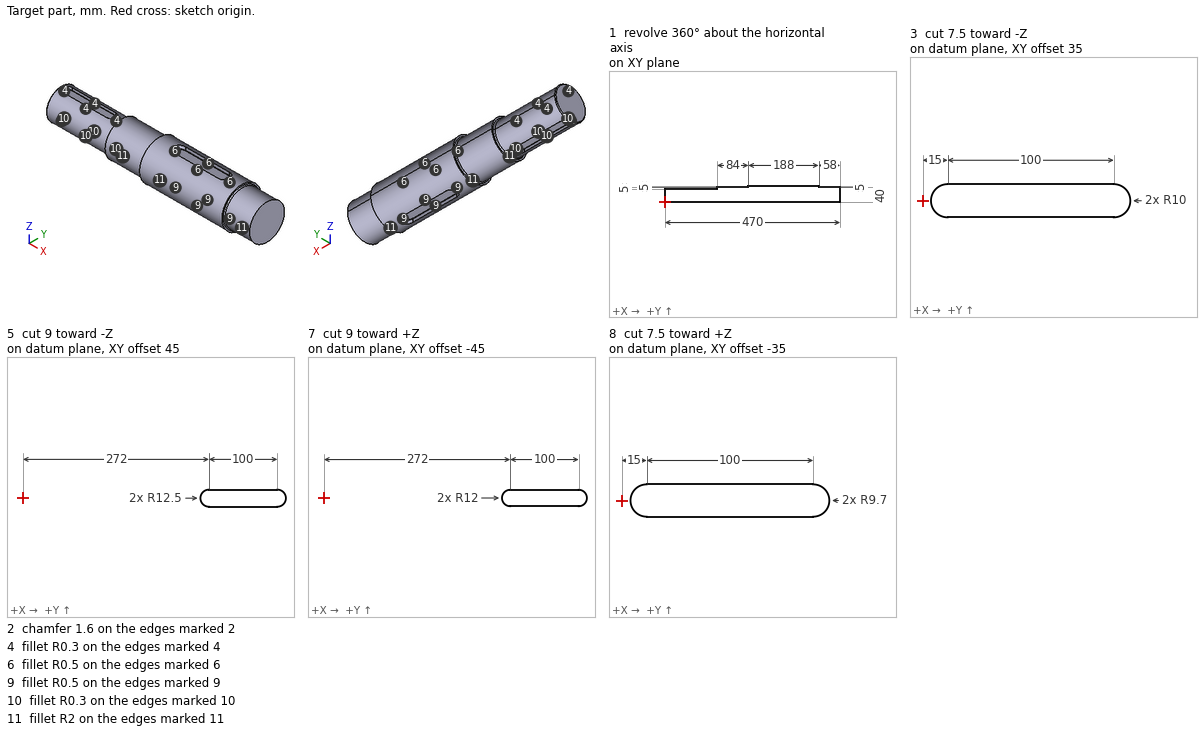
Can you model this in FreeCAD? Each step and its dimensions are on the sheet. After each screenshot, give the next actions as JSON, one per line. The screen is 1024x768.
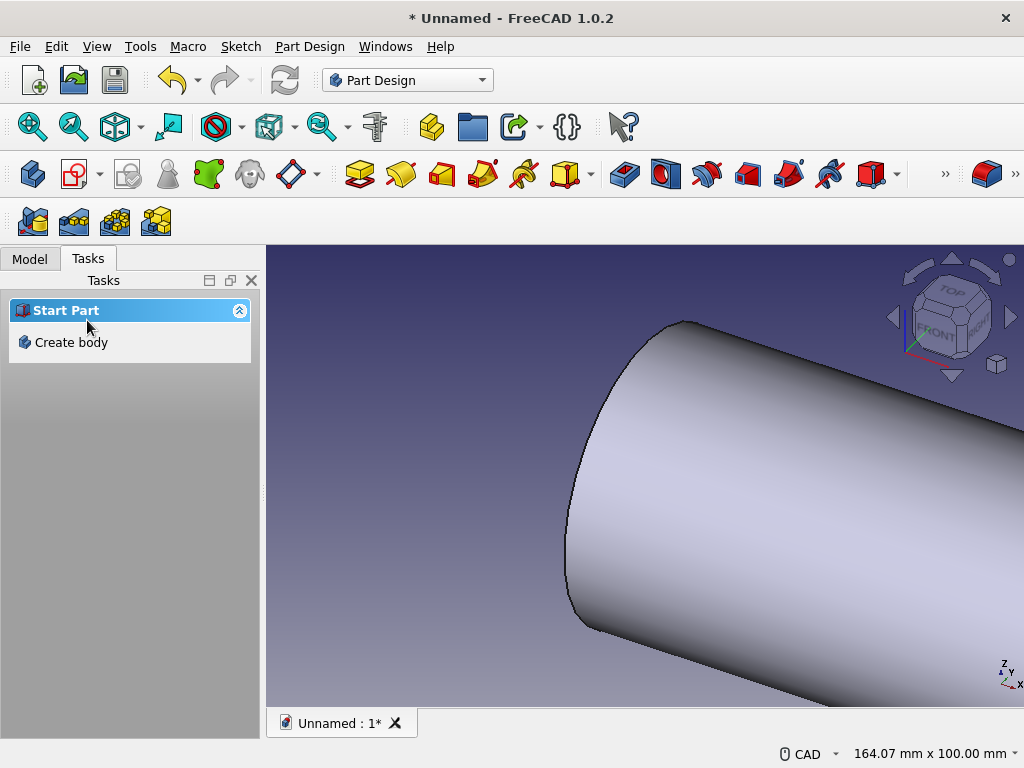
{"action": "left_click", "coordinate": [33, 128]}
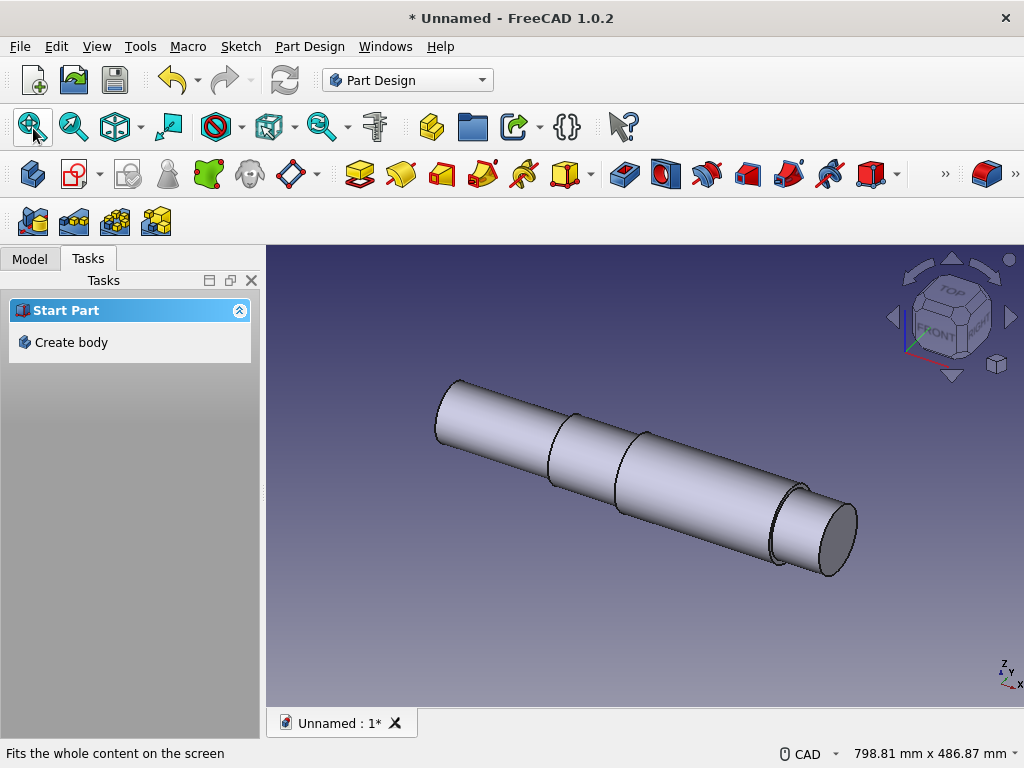
{"action": "left_click", "coordinate": [435, 428]}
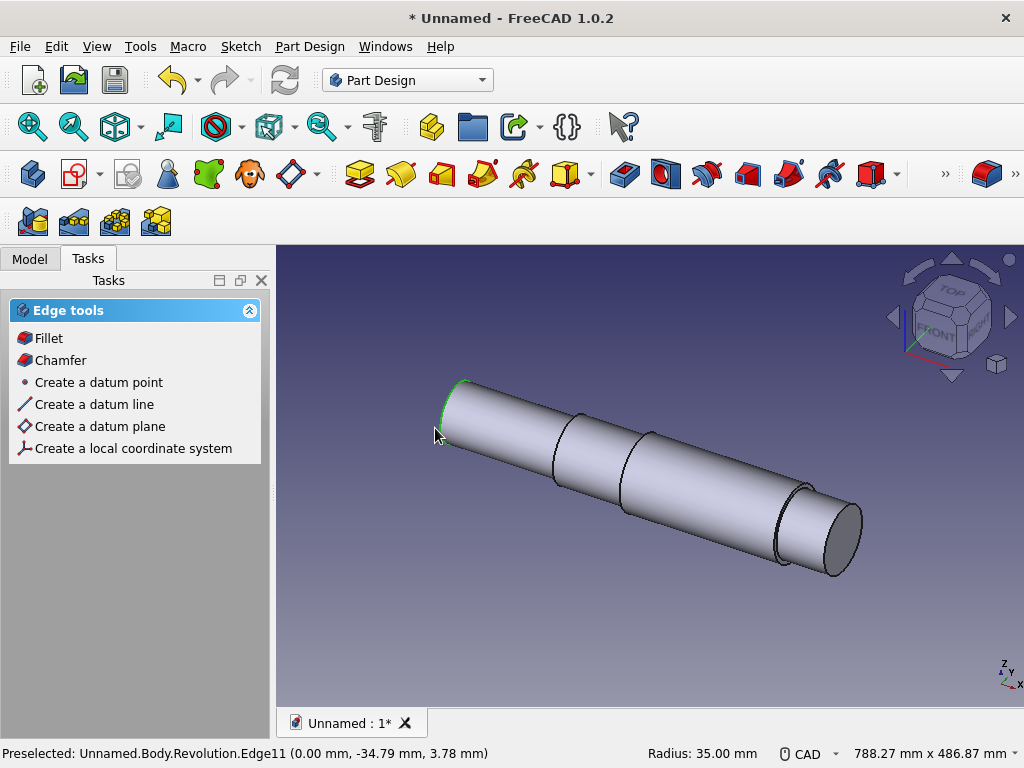
{"action": "left_click", "coordinate": [135, 360]}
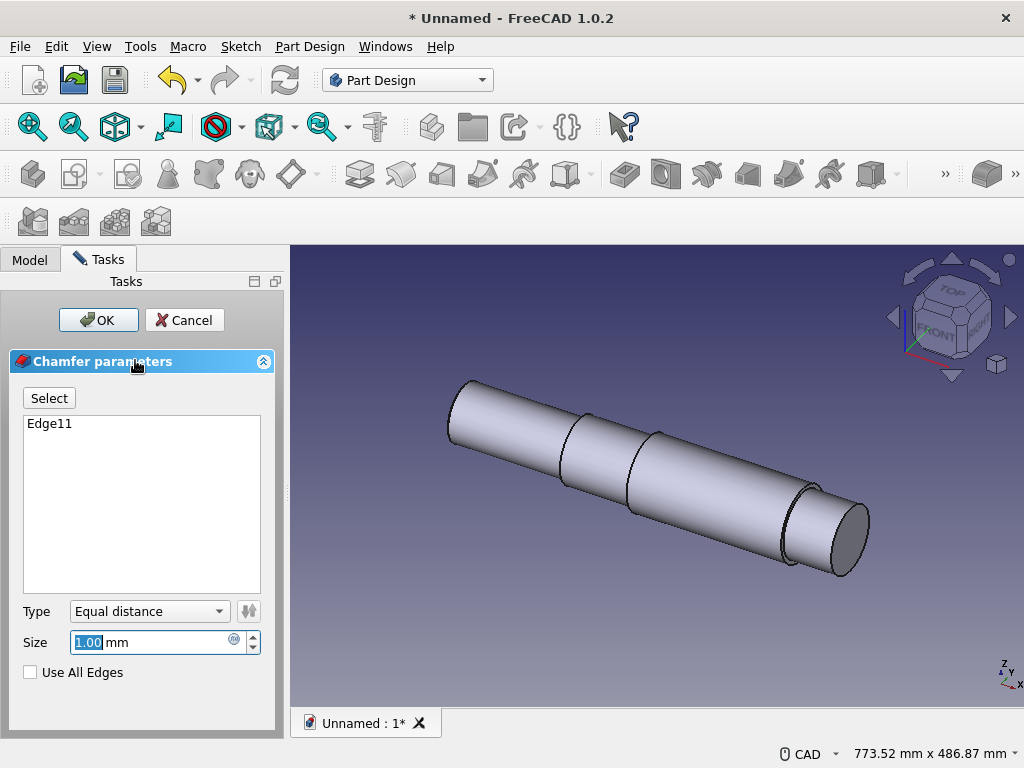
{"action": "type", "text": "1.6"}
{"action": "key", "text": "Tab"}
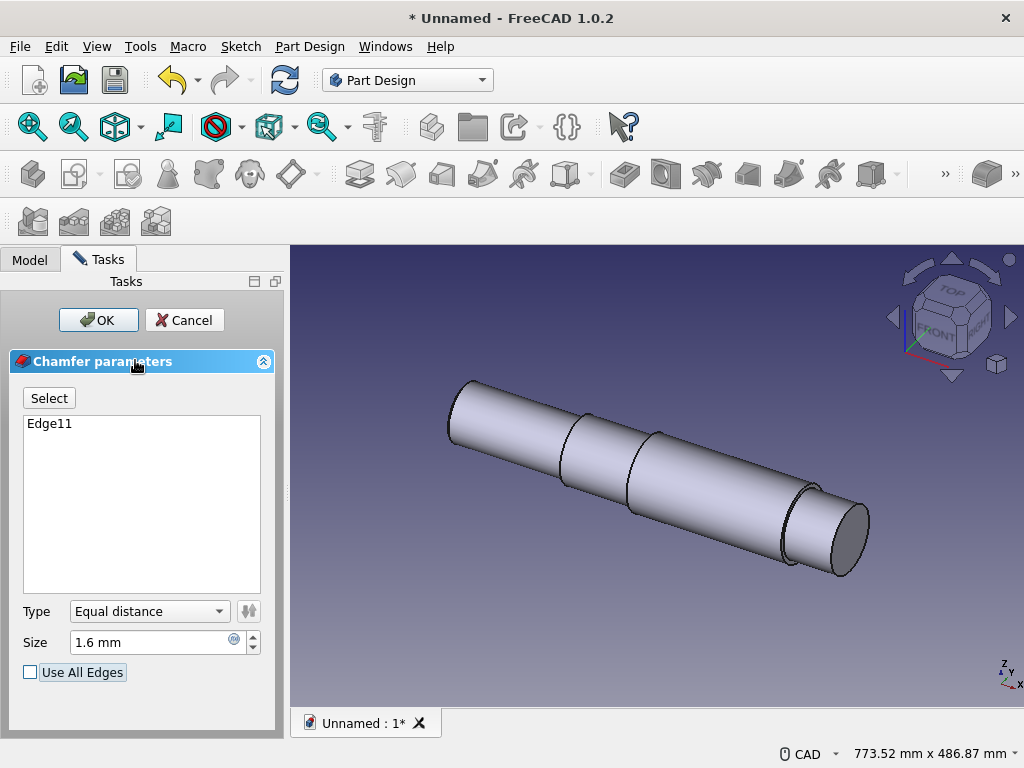
{"action": "left_click", "coordinate": [99, 320]}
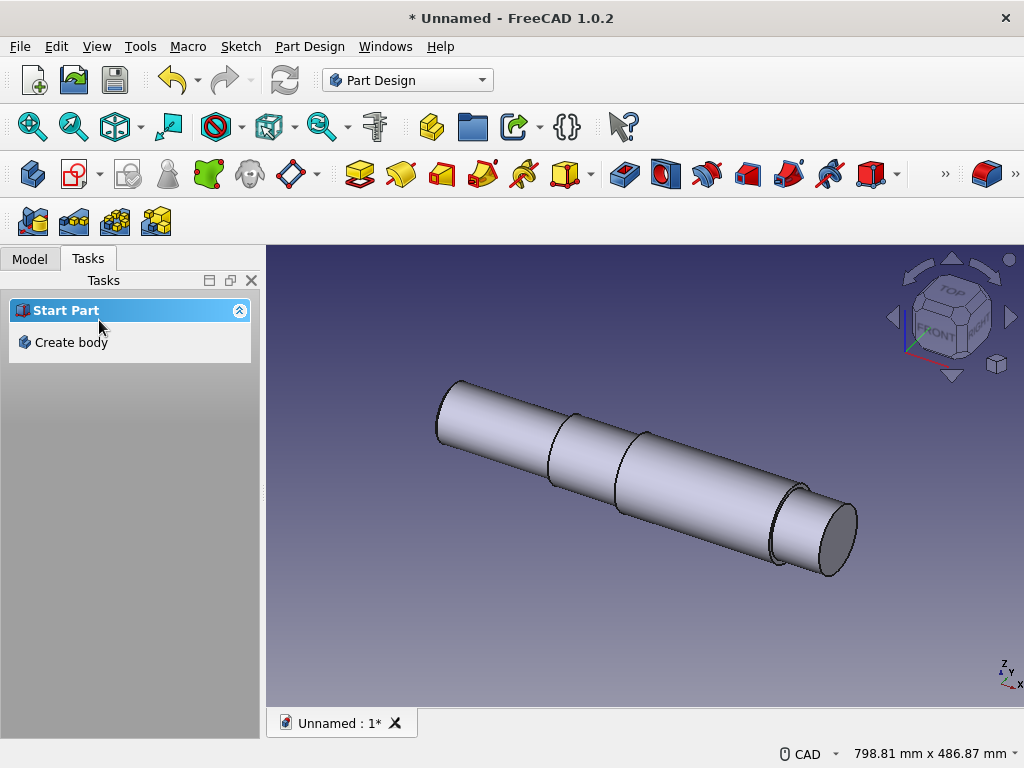
{"action": "left_click", "coordinate": [30, 258]}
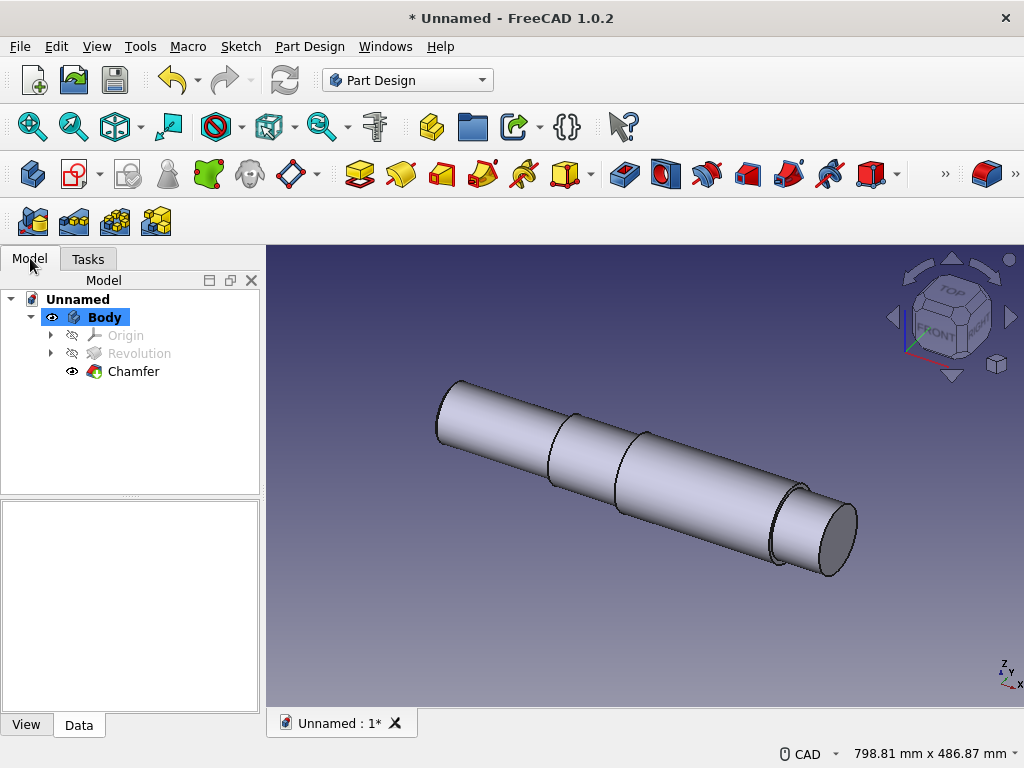
{"action": "left_click", "coordinate": [51, 335]}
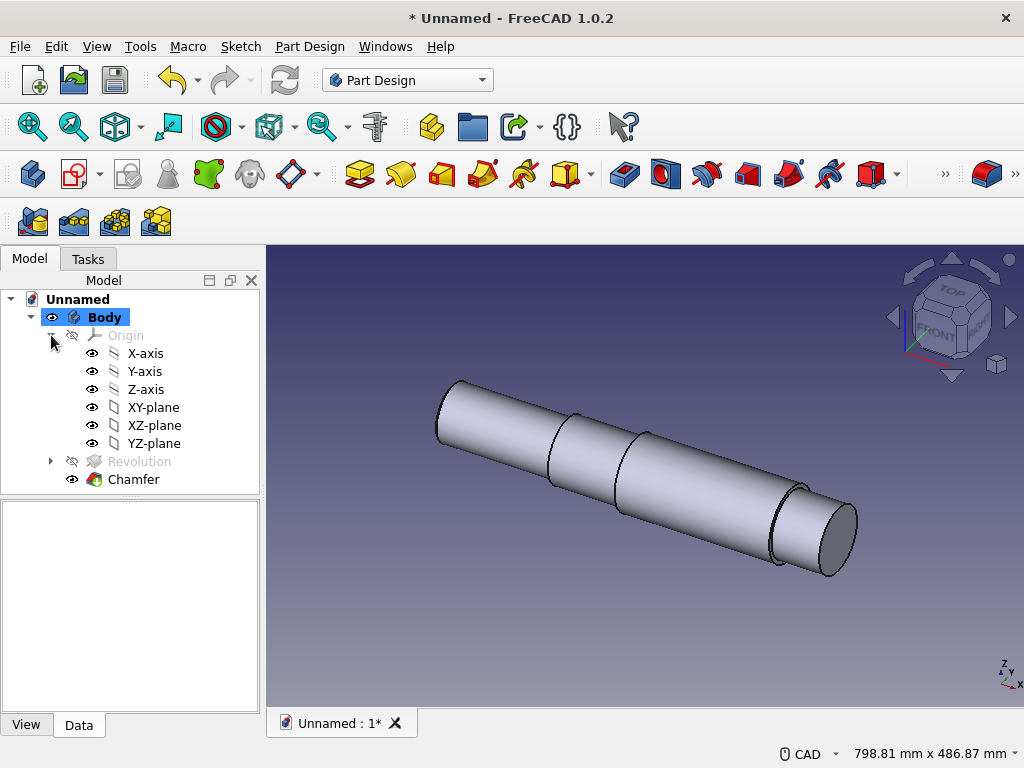
{"action": "left_click", "coordinate": [137, 407]}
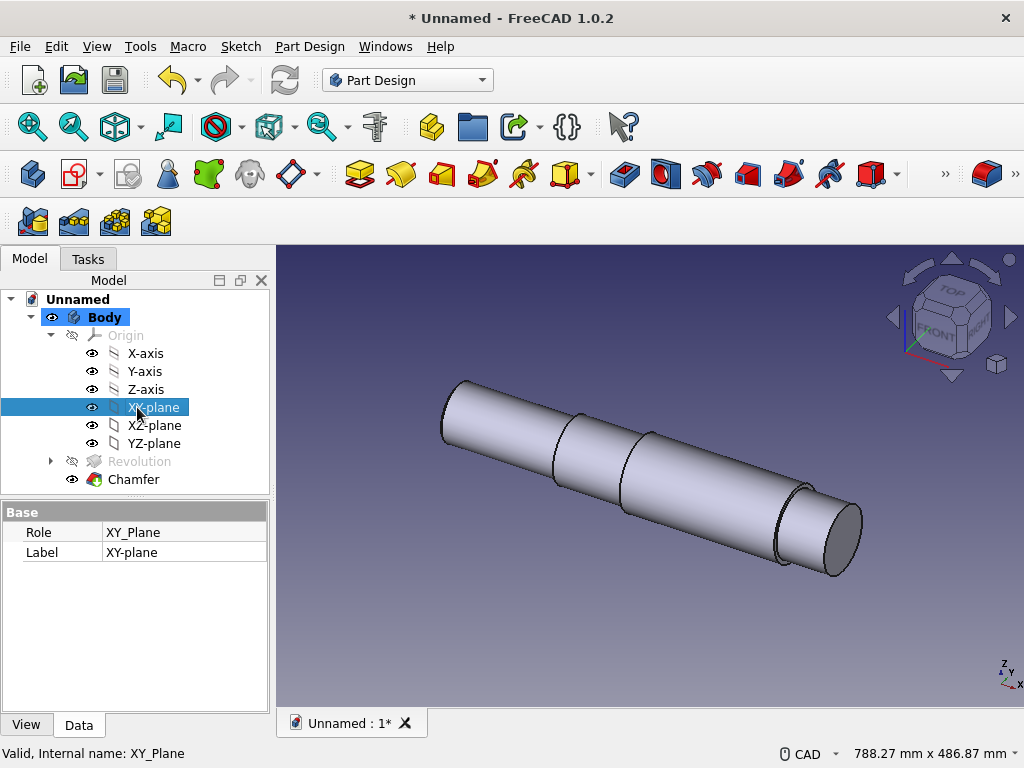
{"action": "left_click", "coordinate": [290, 174]}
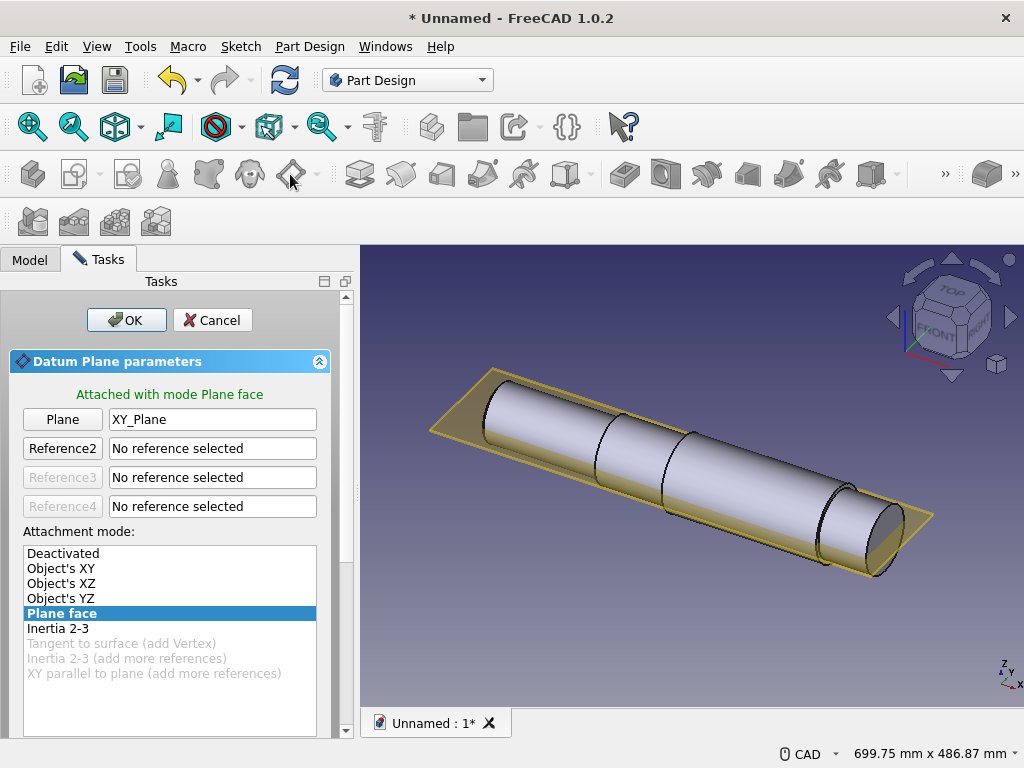
{"action": "scroll", "coordinate": [346, 514], "scroll_direction": "down", "scroll_amount": 4}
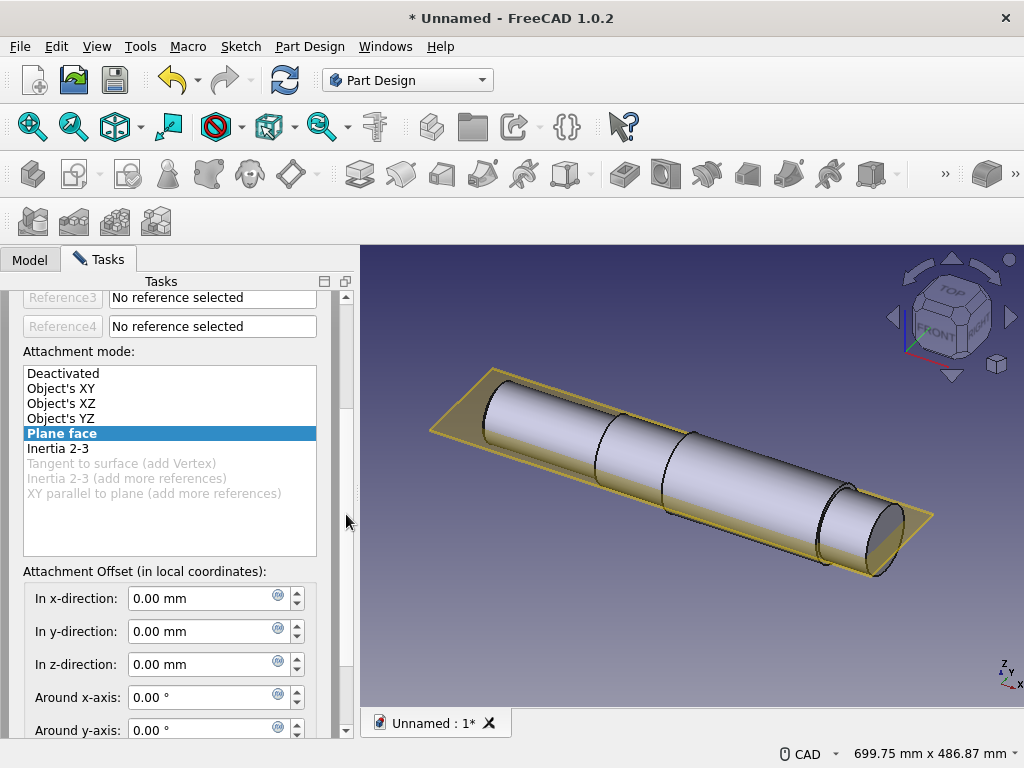
{"action": "triple_click", "coordinate": [210, 604]}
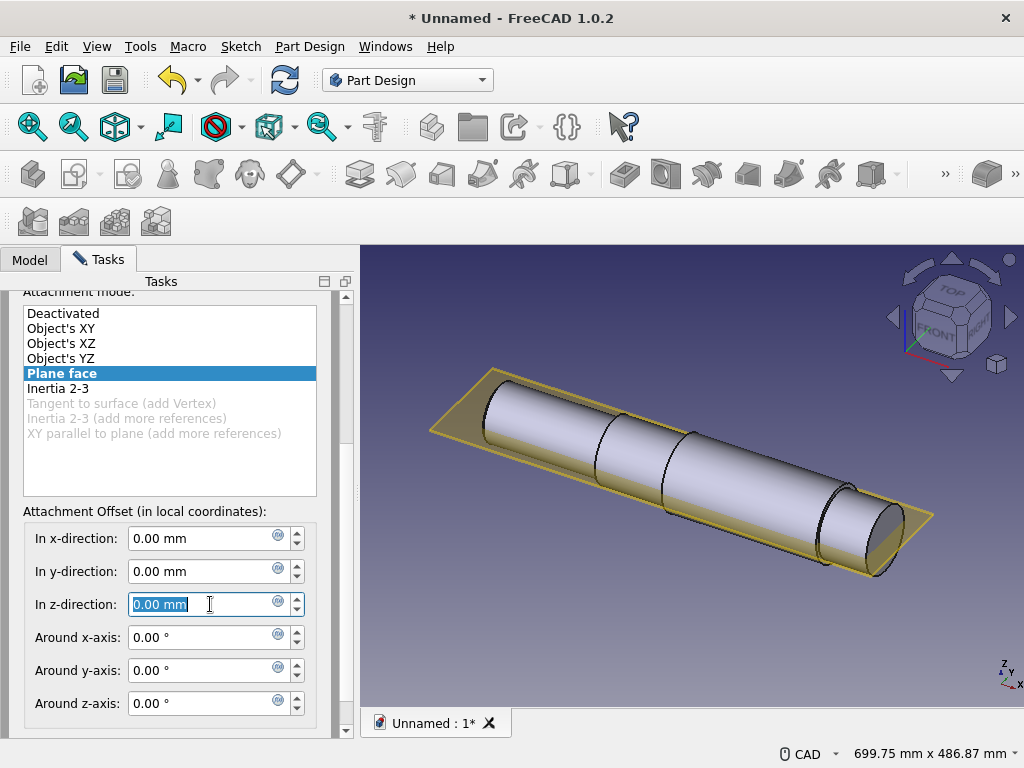
{"action": "type", "text": "35"}
{"action": "key", "text": "Tab"}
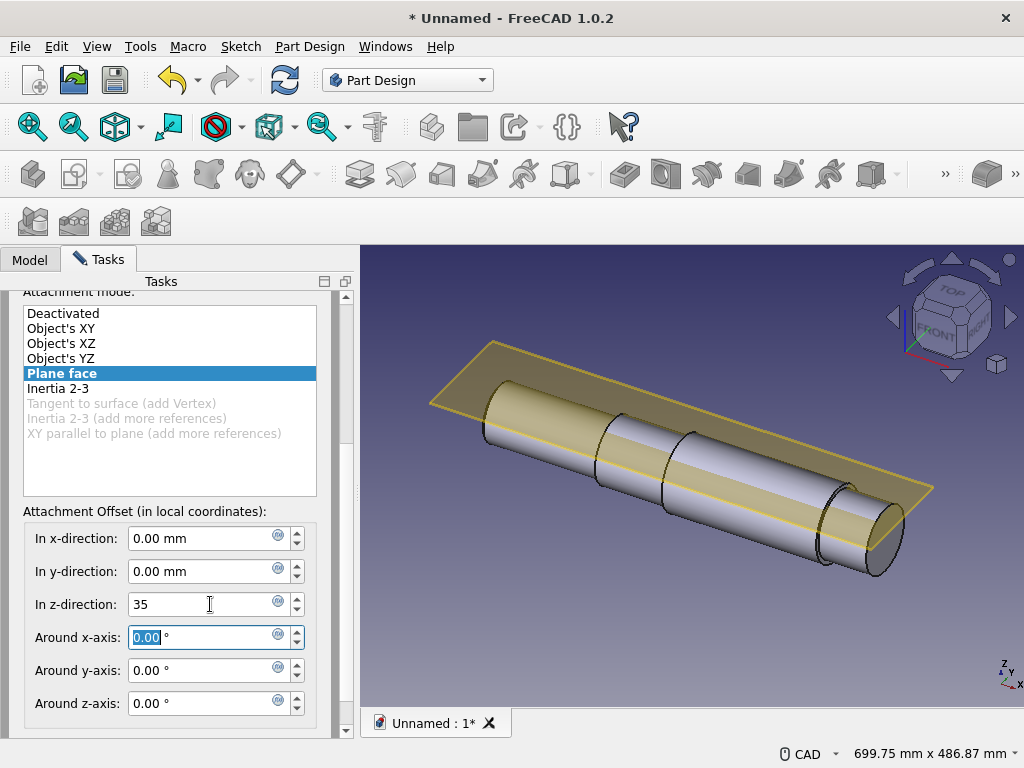
{"action": "scroll", "coordinate": [346, 514], "scroll_direction": "up", "scroll_amount": 5}